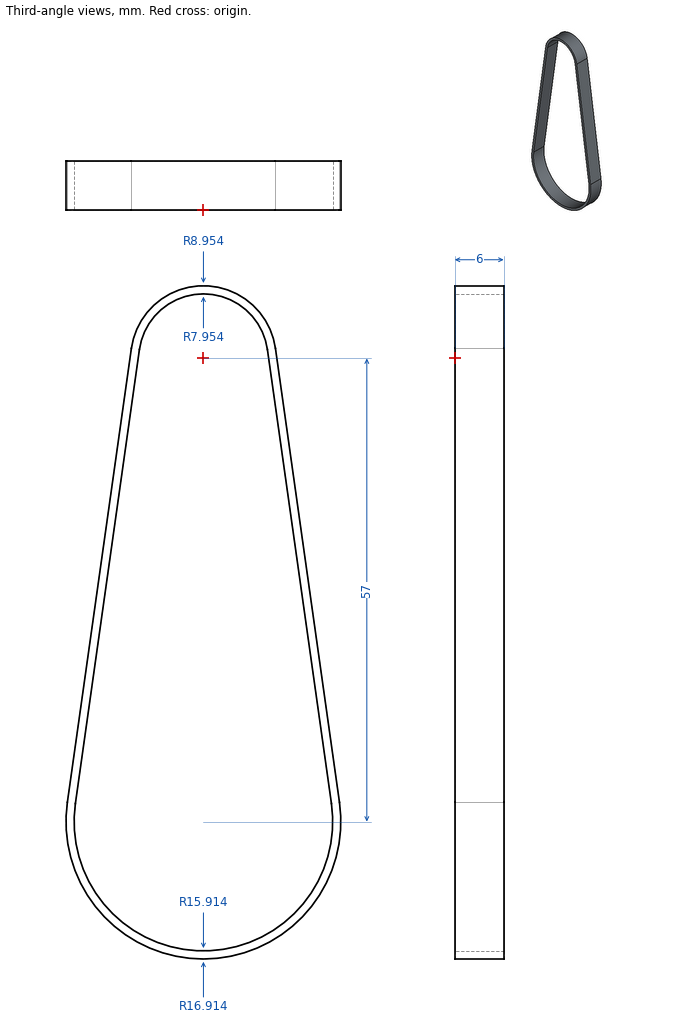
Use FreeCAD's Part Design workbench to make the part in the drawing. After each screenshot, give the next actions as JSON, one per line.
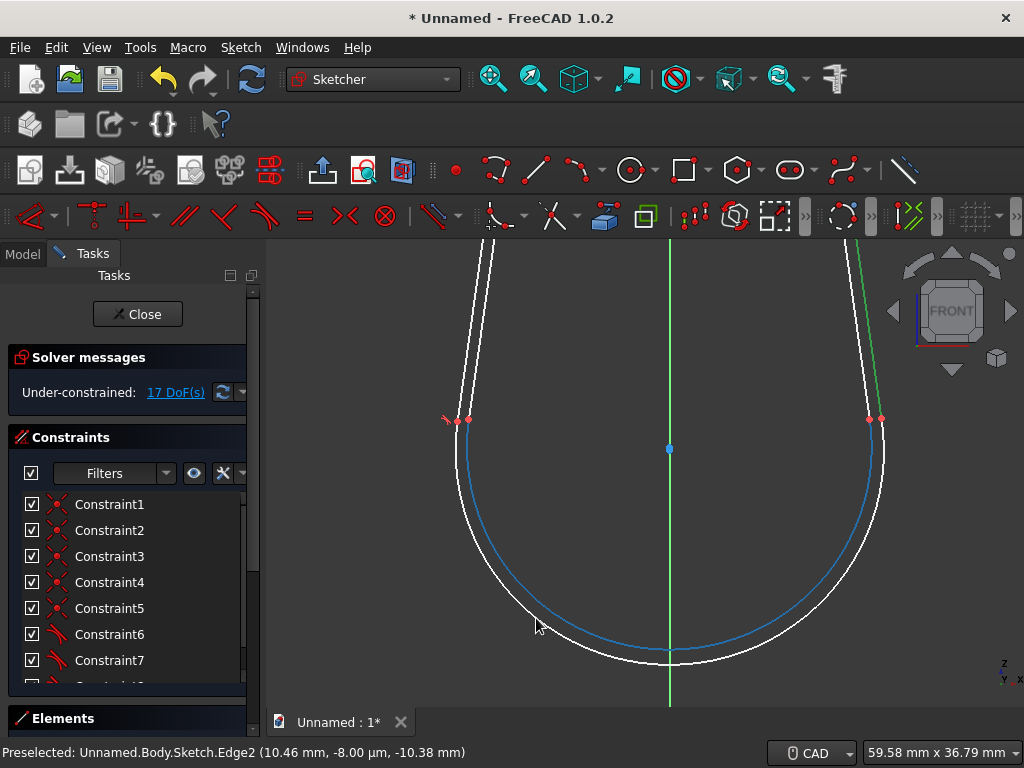
{"action": "left_click", "coordinate": [535, 617]}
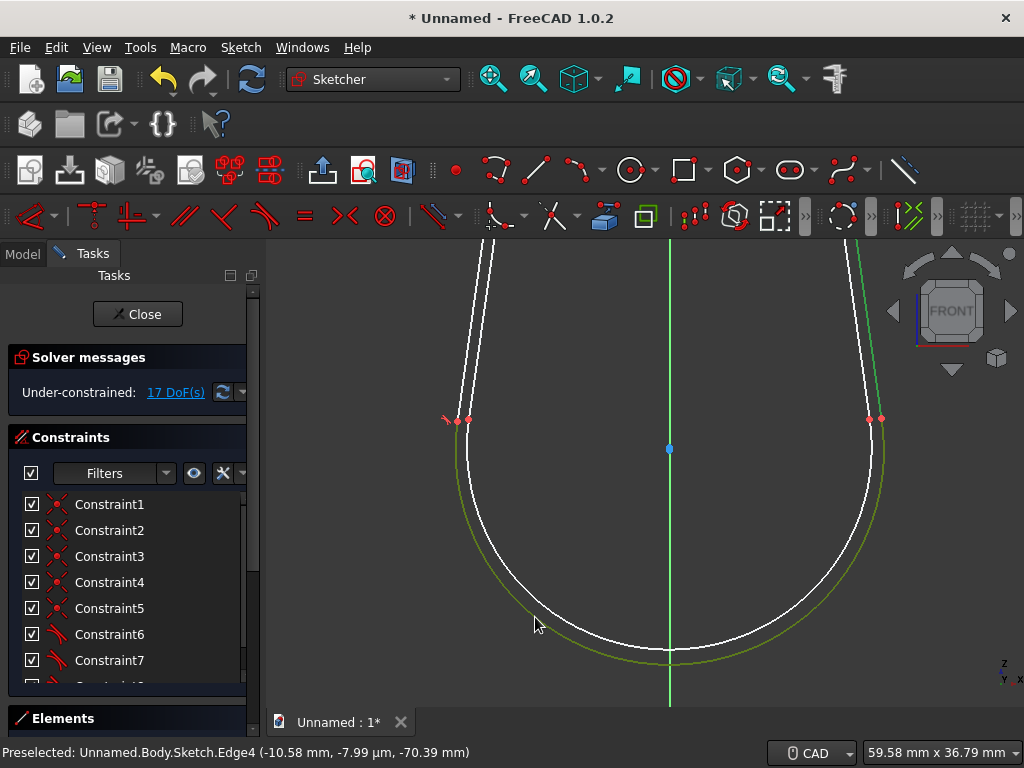
{"action": "left_click", "coordinate": [266, 216]}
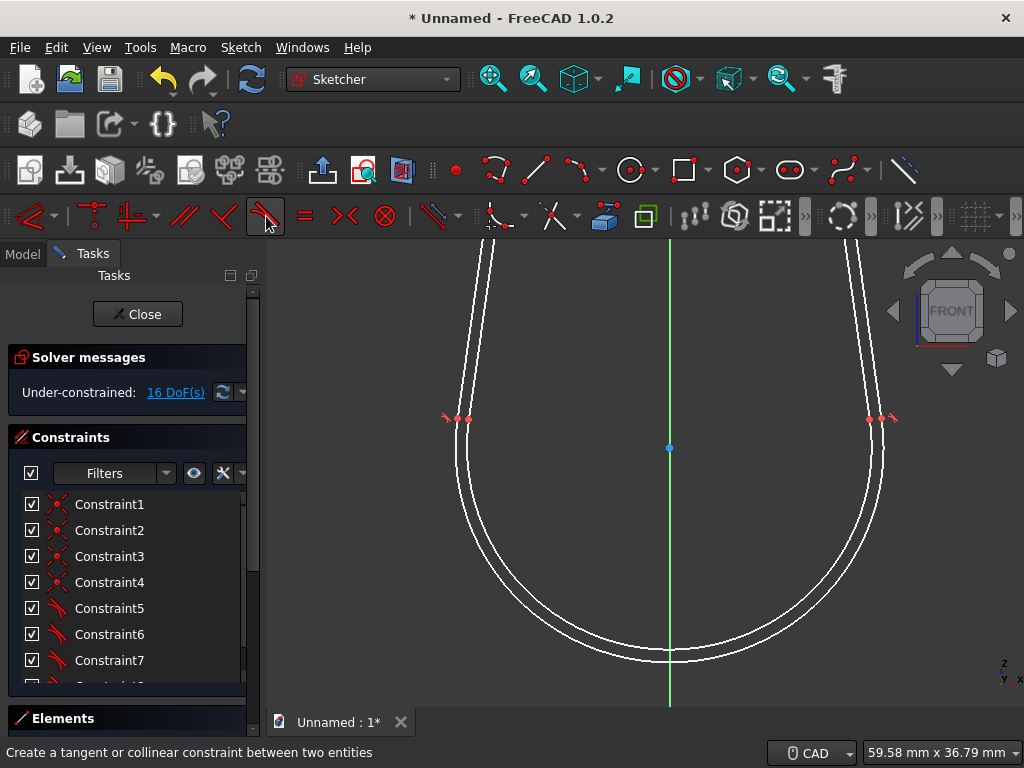
{"action": "left_click", "coordinate": [489, 277]}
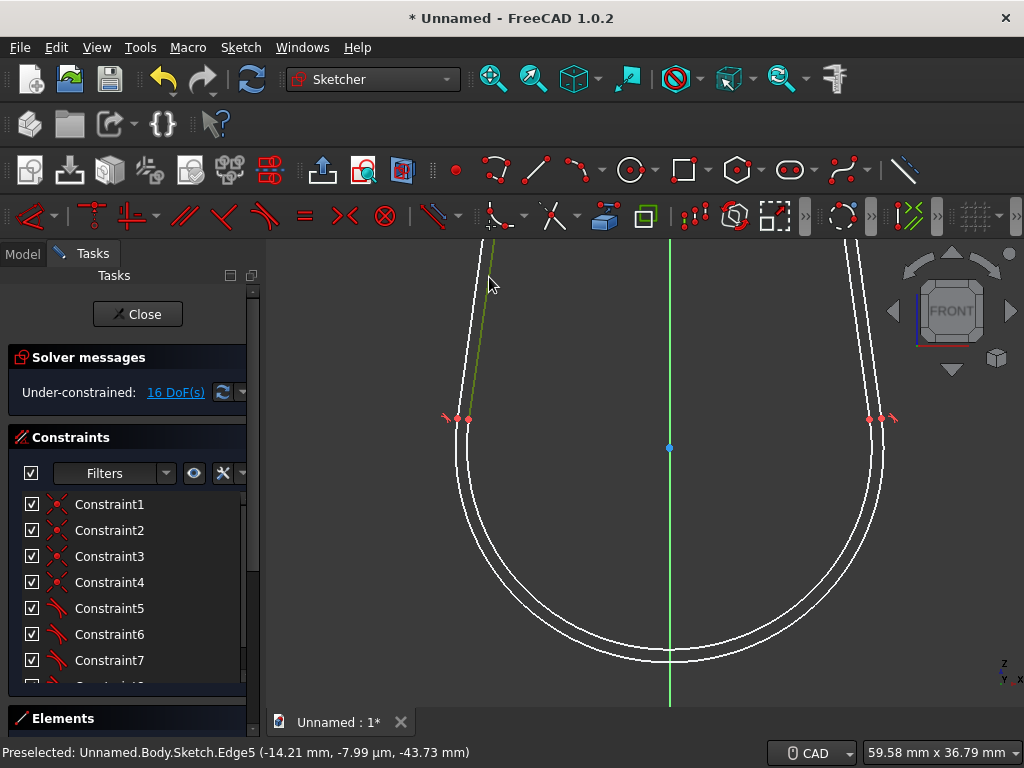
{"action": "left_click", "coordinate": [541, 604]}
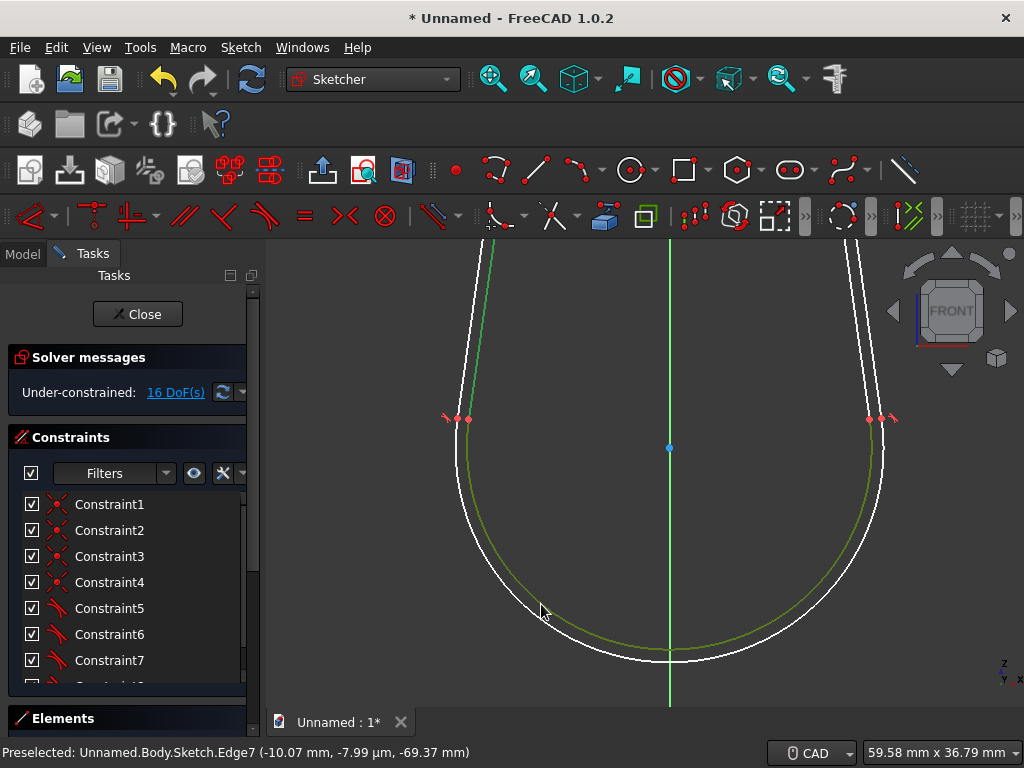
{"action": "left_click", "coordinate": [266, 216]}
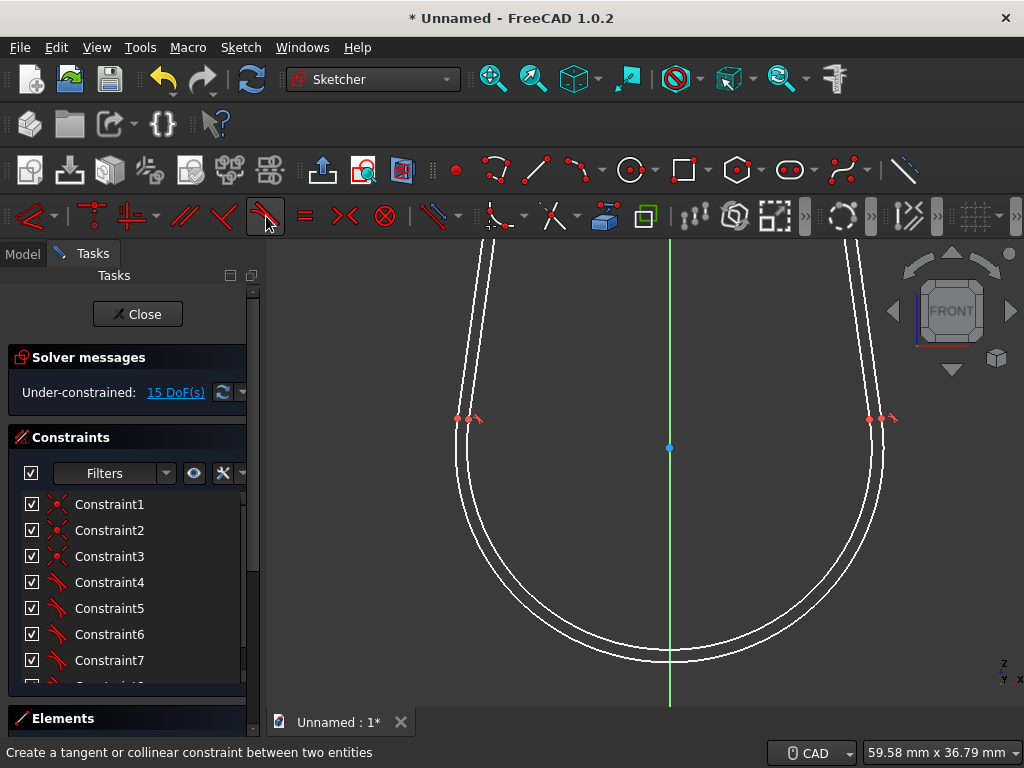
{"action": "left_click", "coordinate": [489, 277]}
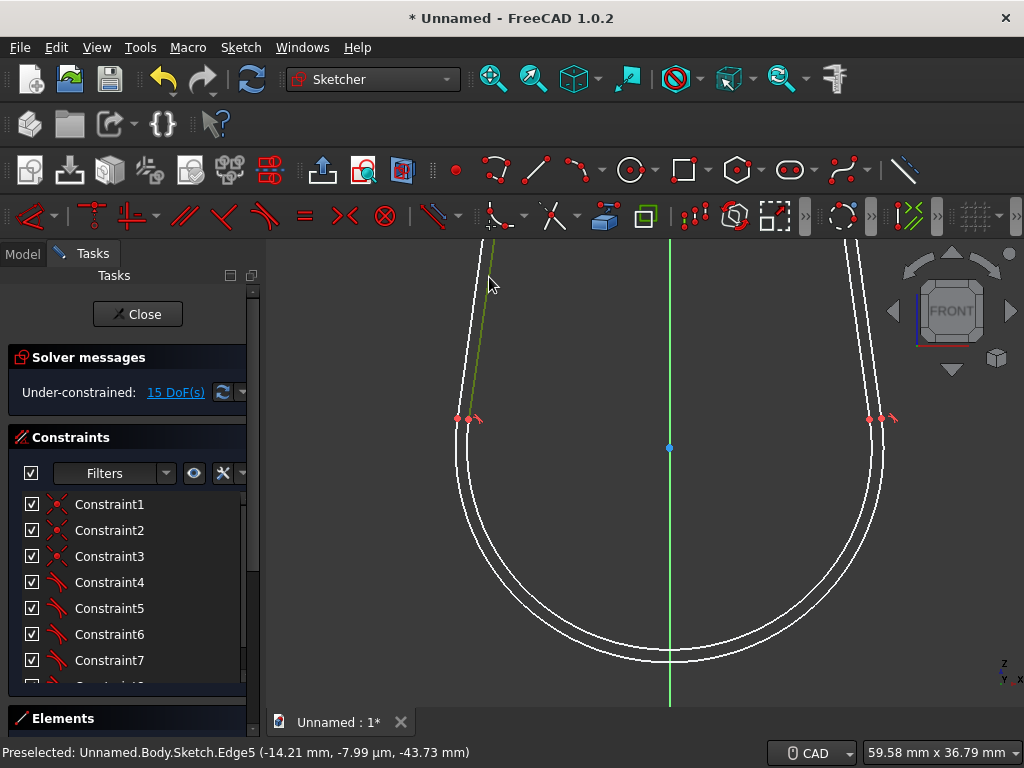
{"action": "scroll", "coordinate": [536, 619], "scroll_direction": "down", "scroll_amount": 6}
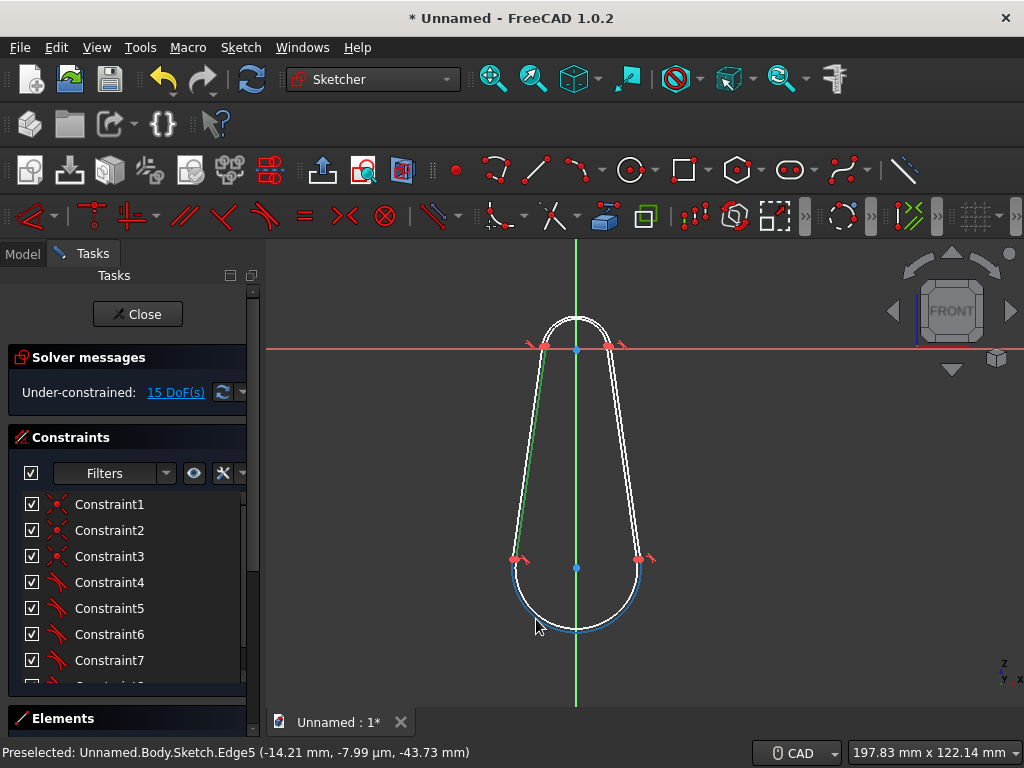
{"action": "scroll", "coordinate": [600, 330], "scroll_direction": "up", "scroll_amount": 8}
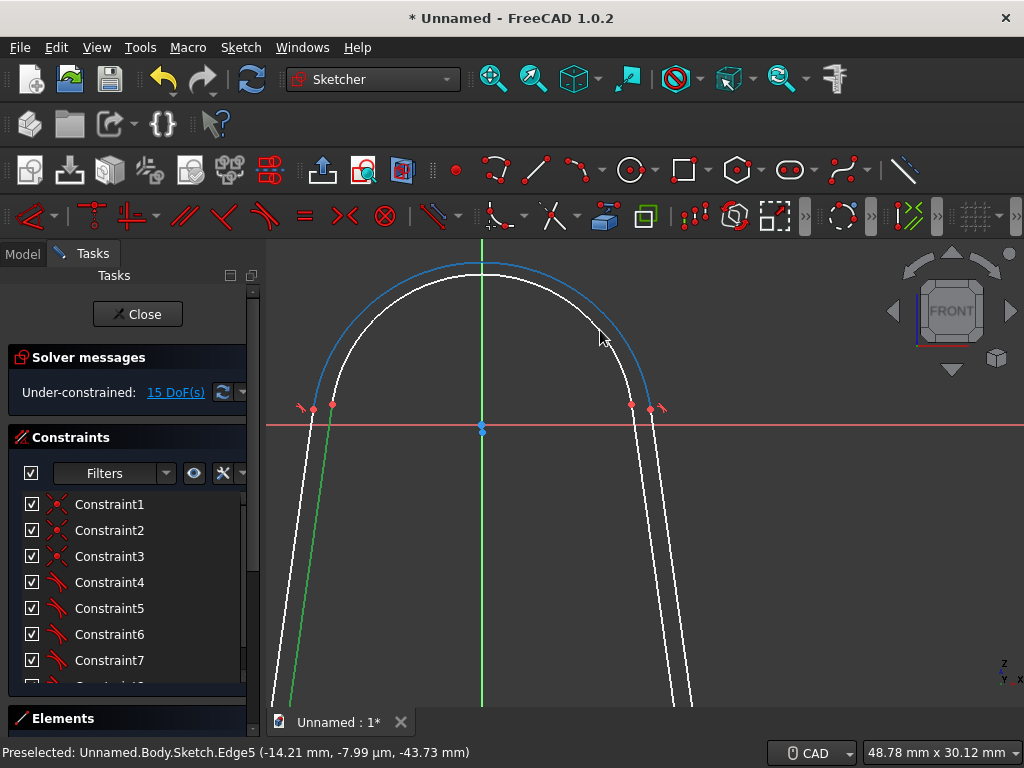
{"action": "left_click", "coordinate": [596, 327]}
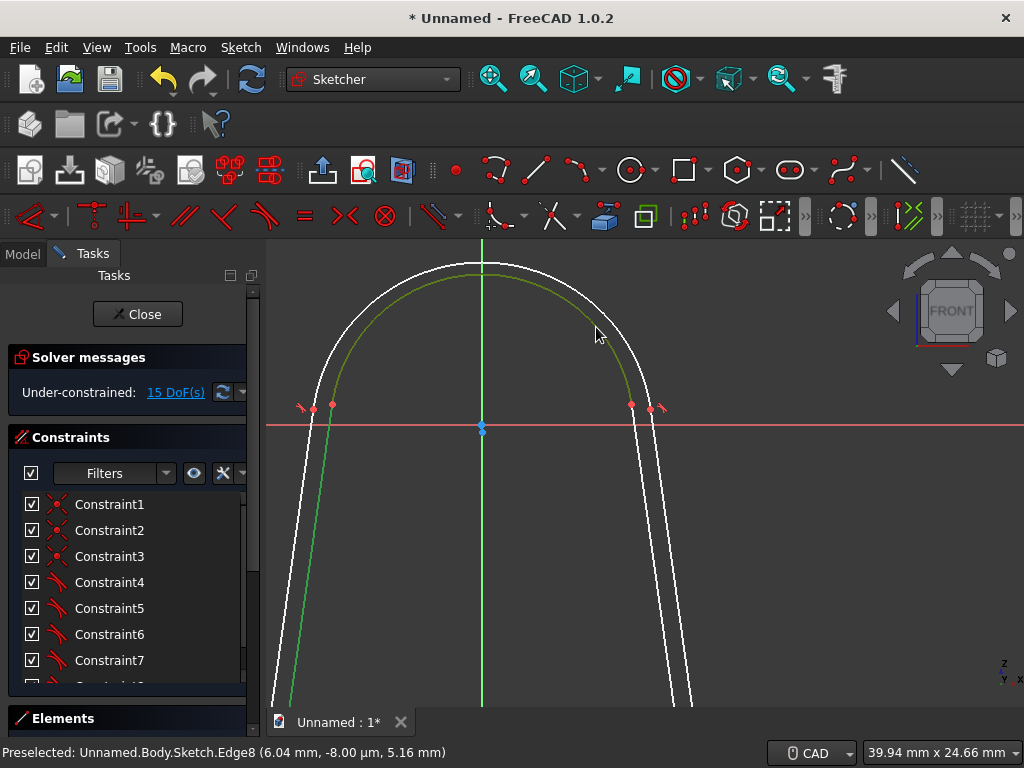
{"action": "left_click", "coordinate": [266, 216]}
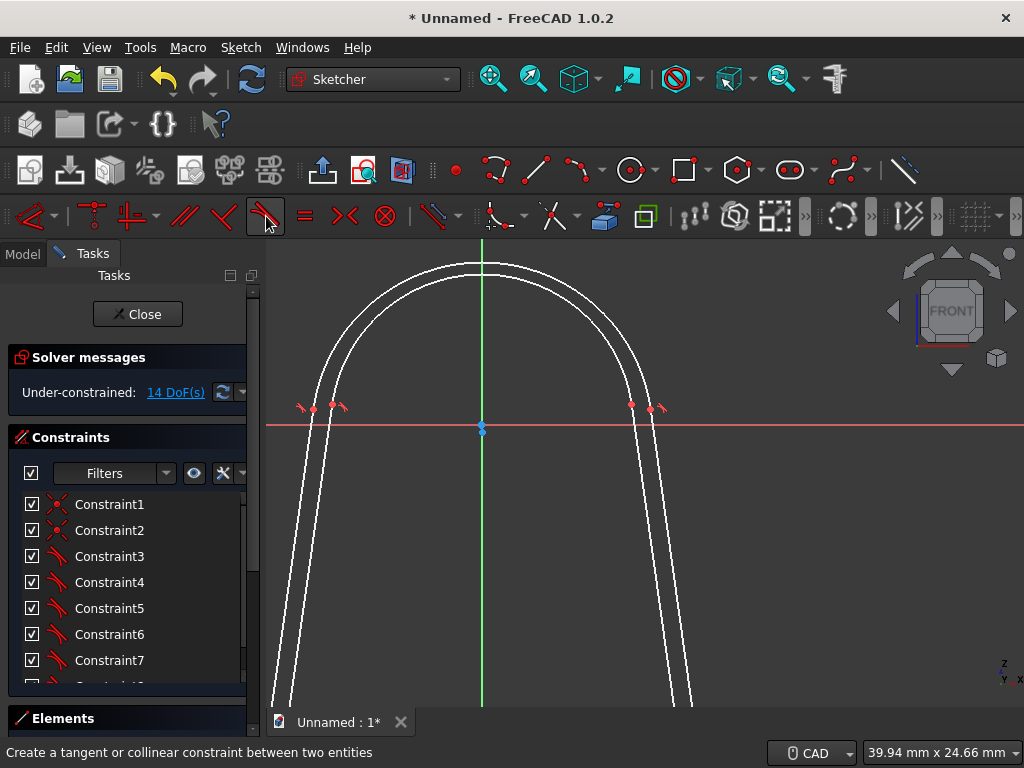
{"action": "left_click", "coordinate": [661, 617]}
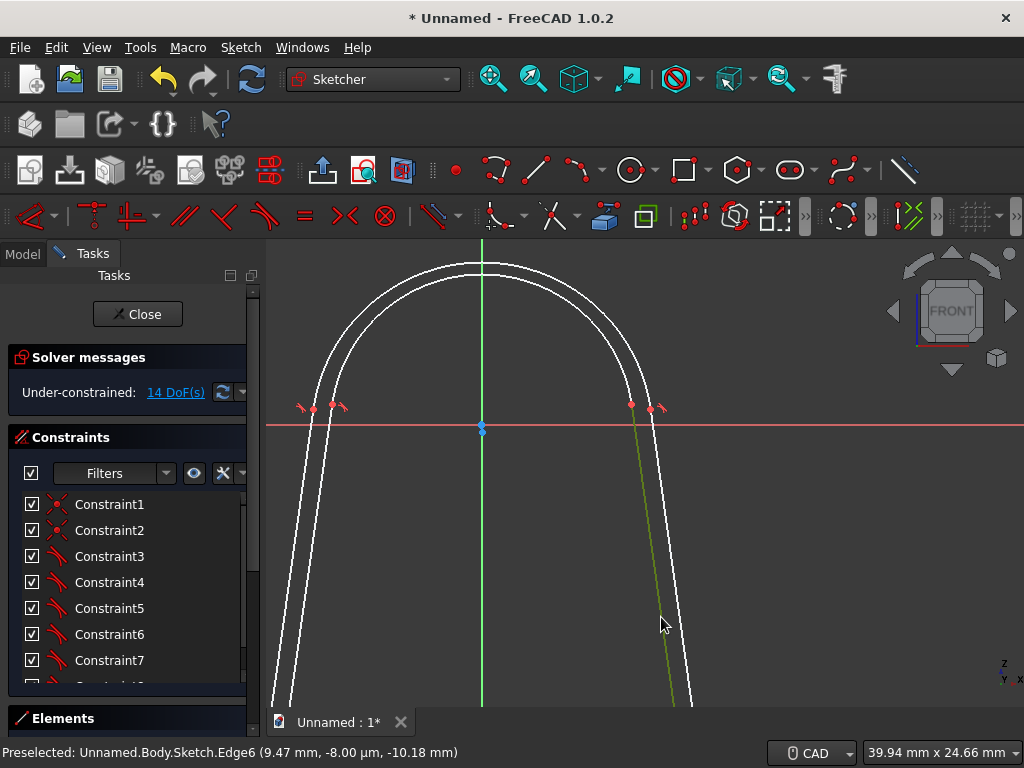
{"action": "scroll", "coordinate": [600, 329], "scroll_direction": "down", "scroll_amount": 8}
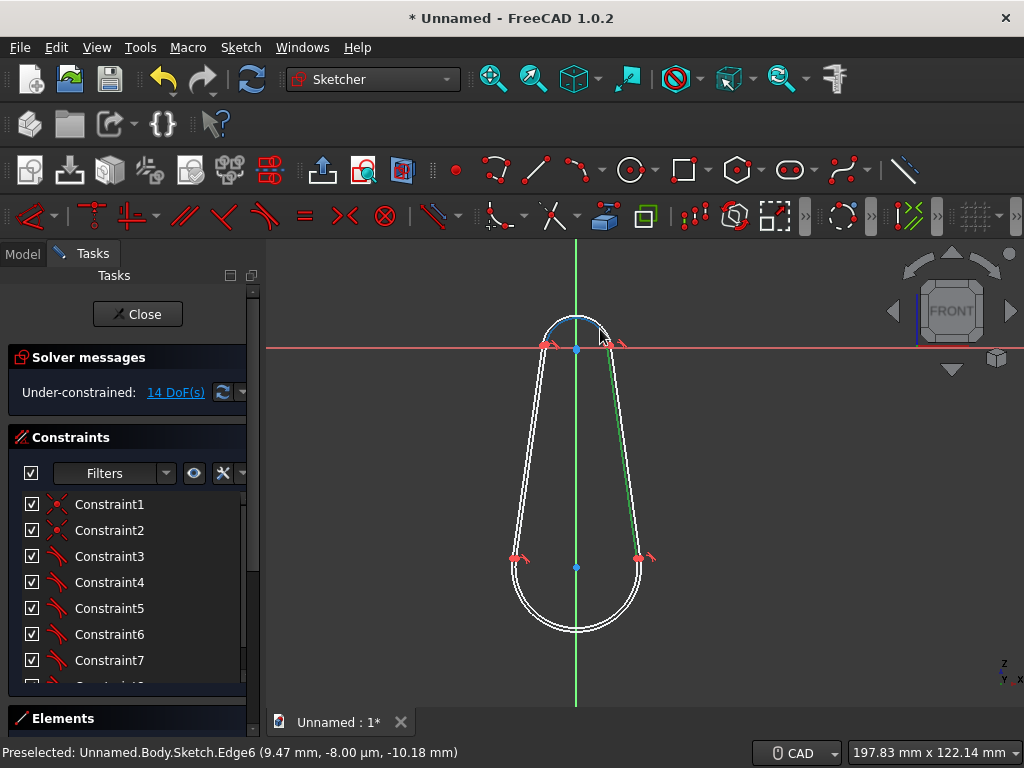
{"action": "scroll", "coordinate": [538, 614], "scroll_direction": "up", "scroll_amount": 7}